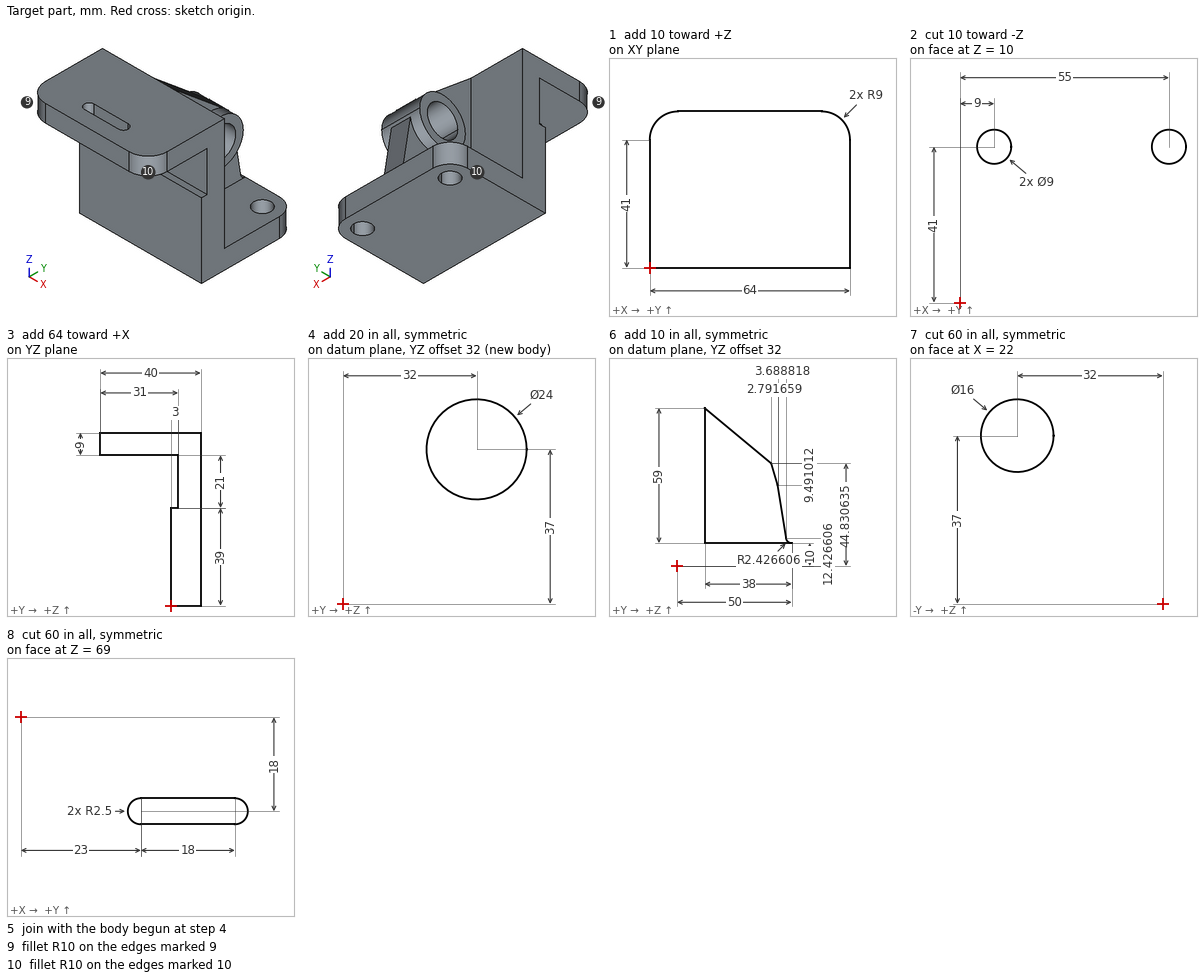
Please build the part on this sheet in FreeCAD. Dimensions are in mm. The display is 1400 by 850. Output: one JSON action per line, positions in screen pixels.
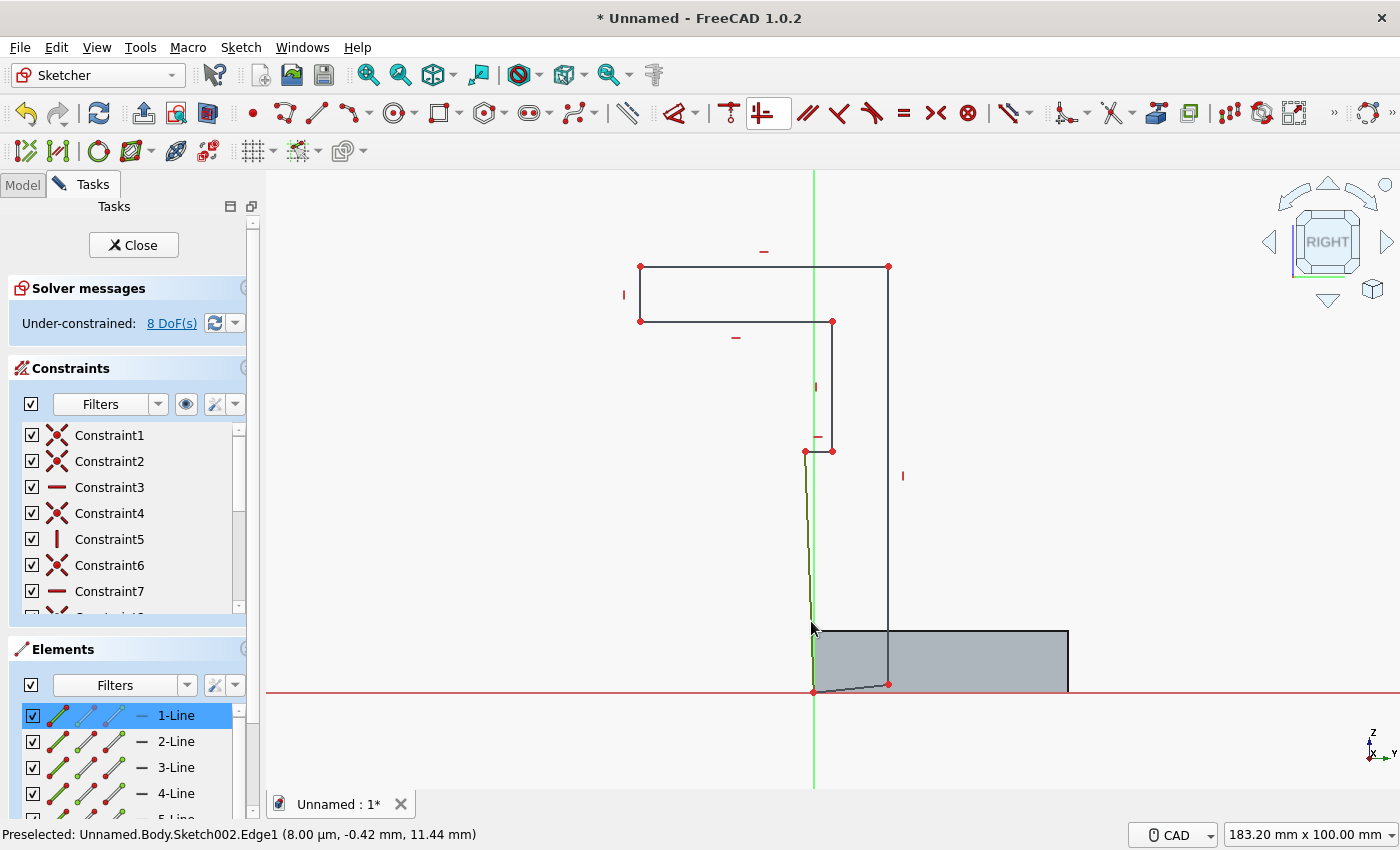
{"action": "key", "text": "v"}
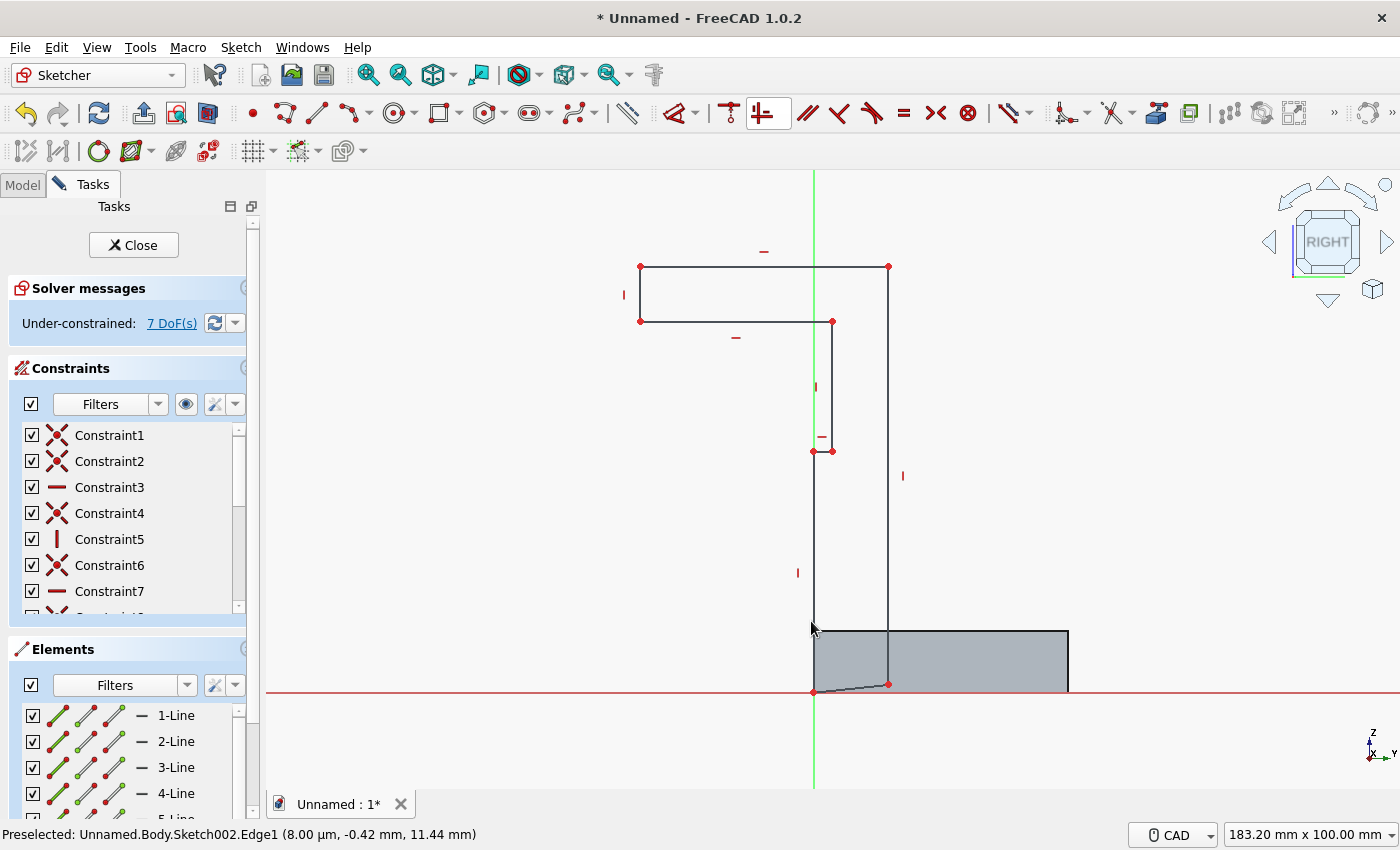
{"action": "left_click", "coordinate": [836, 690]}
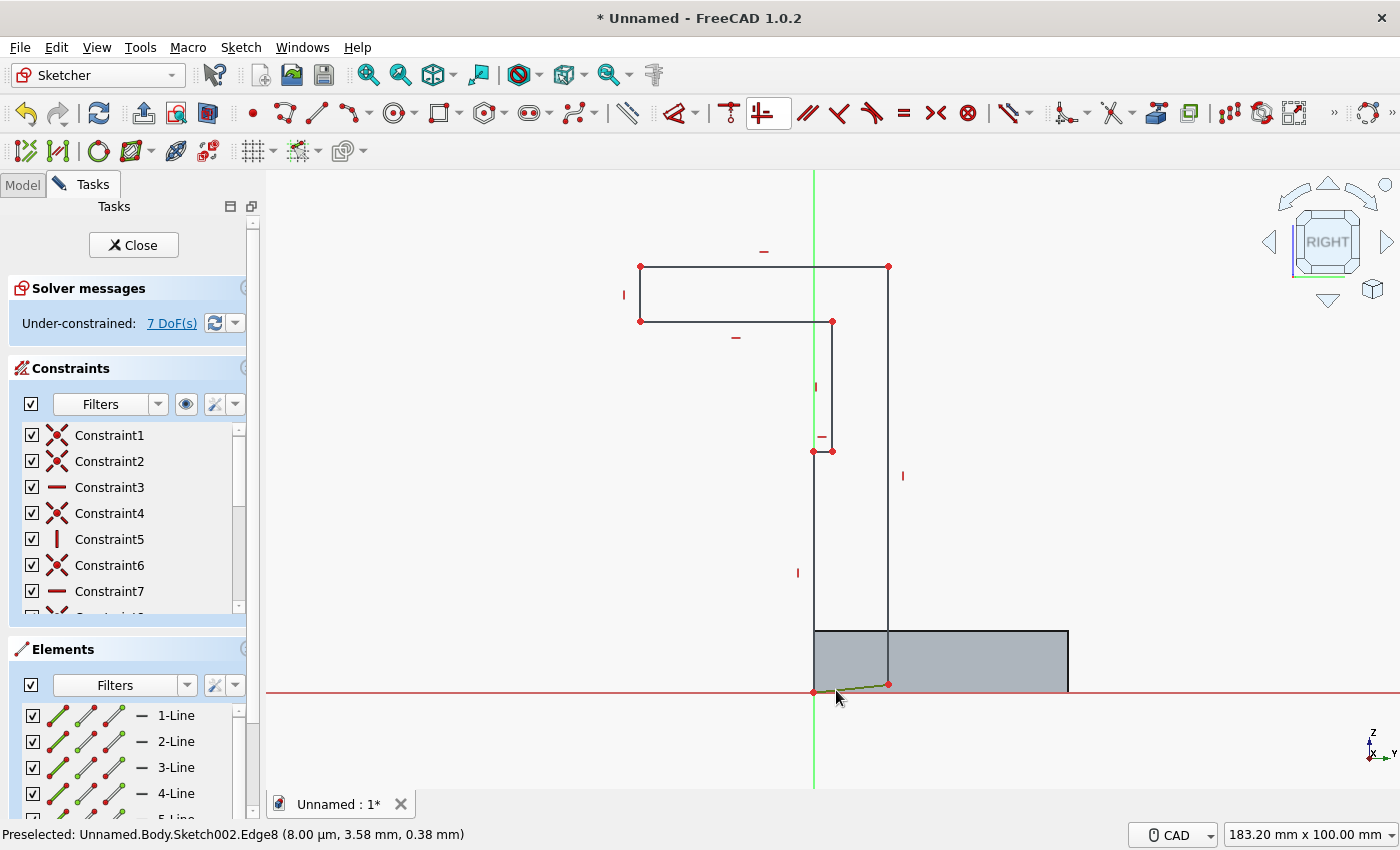
{"action": "key", "text": "h"}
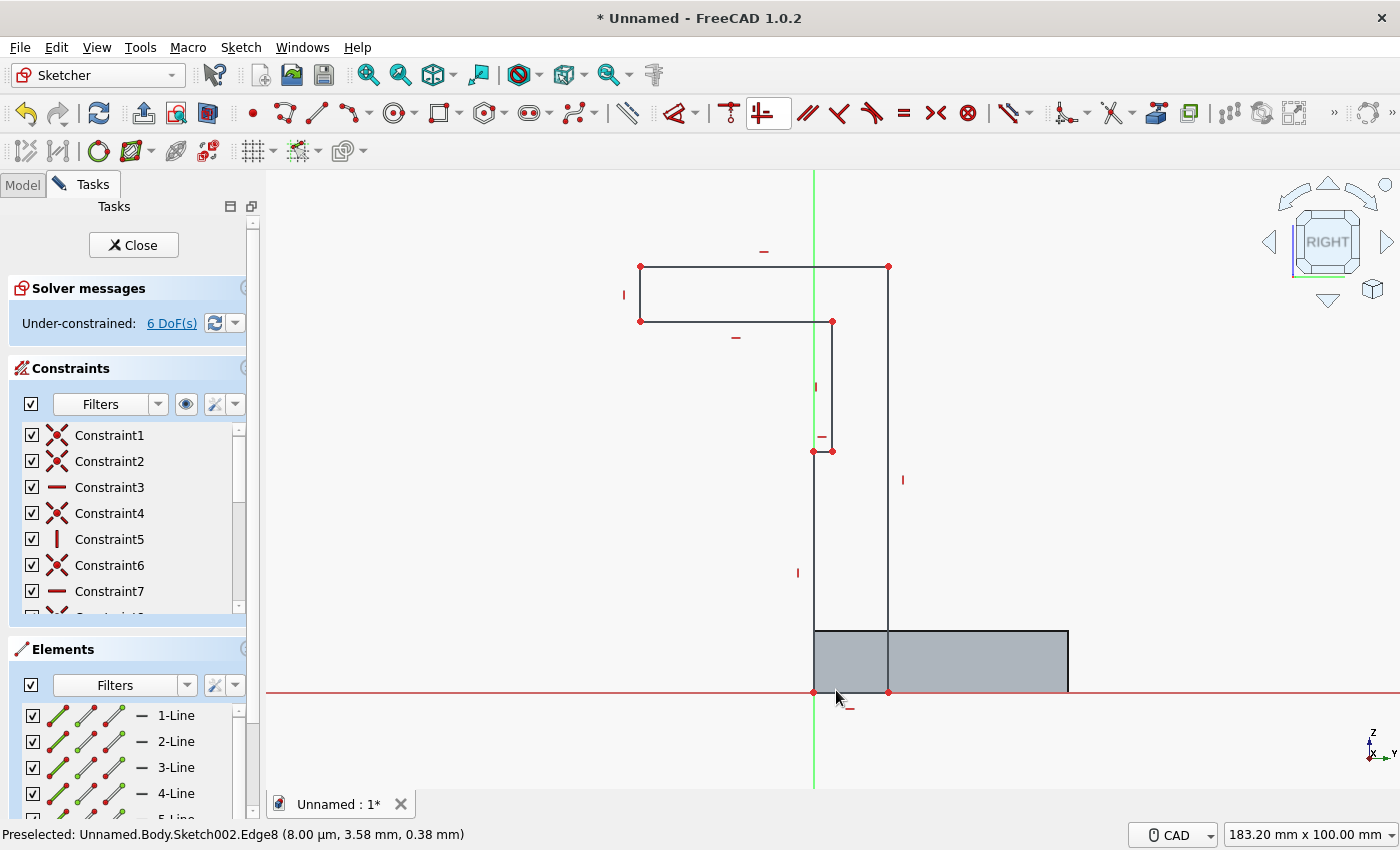
{"action": "left_click", "coordinate": [674, 114]}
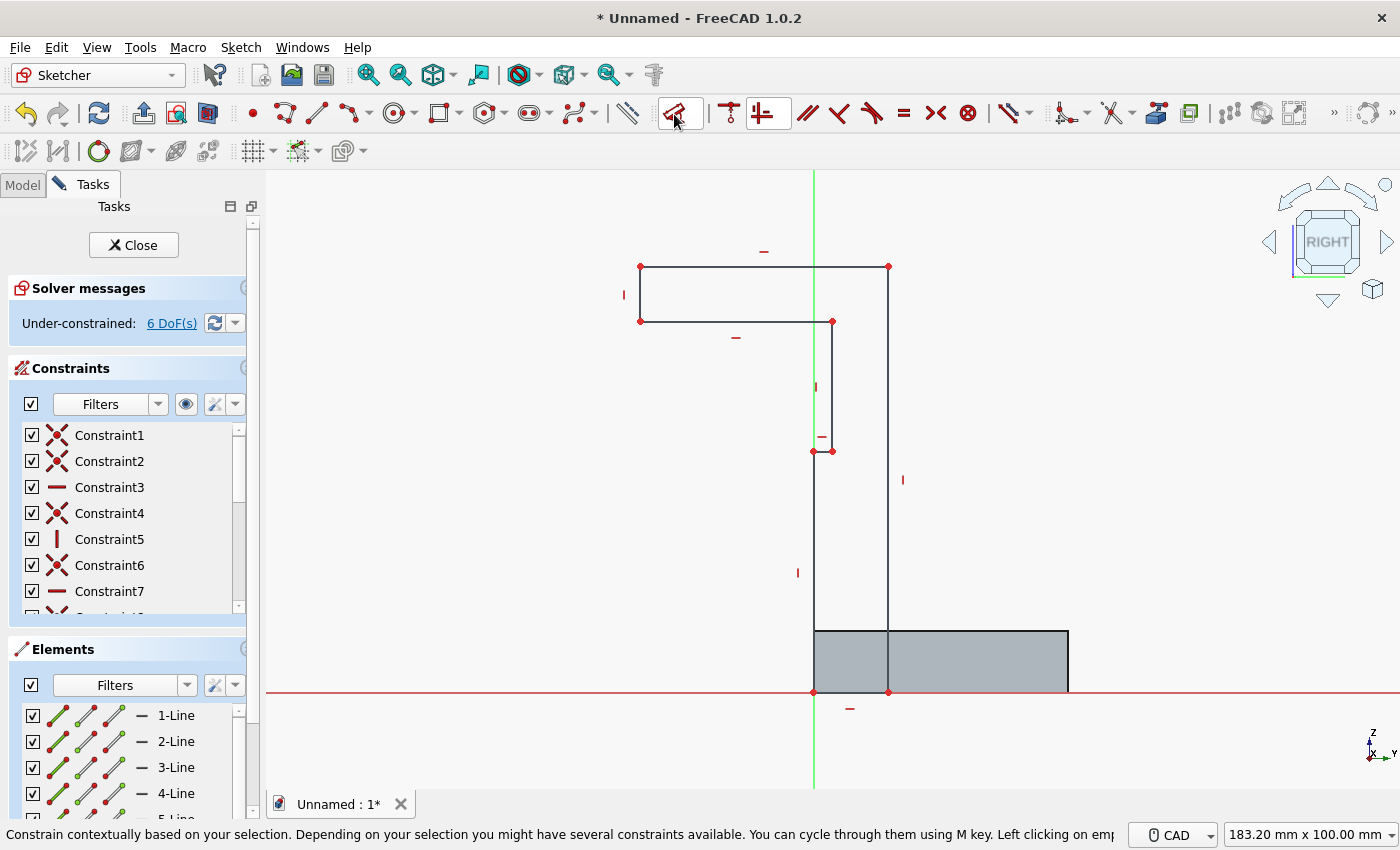
{"action": "scroll", "coordinate": [823, 452], "scroll_direction": "up", "scroll_amount": 4}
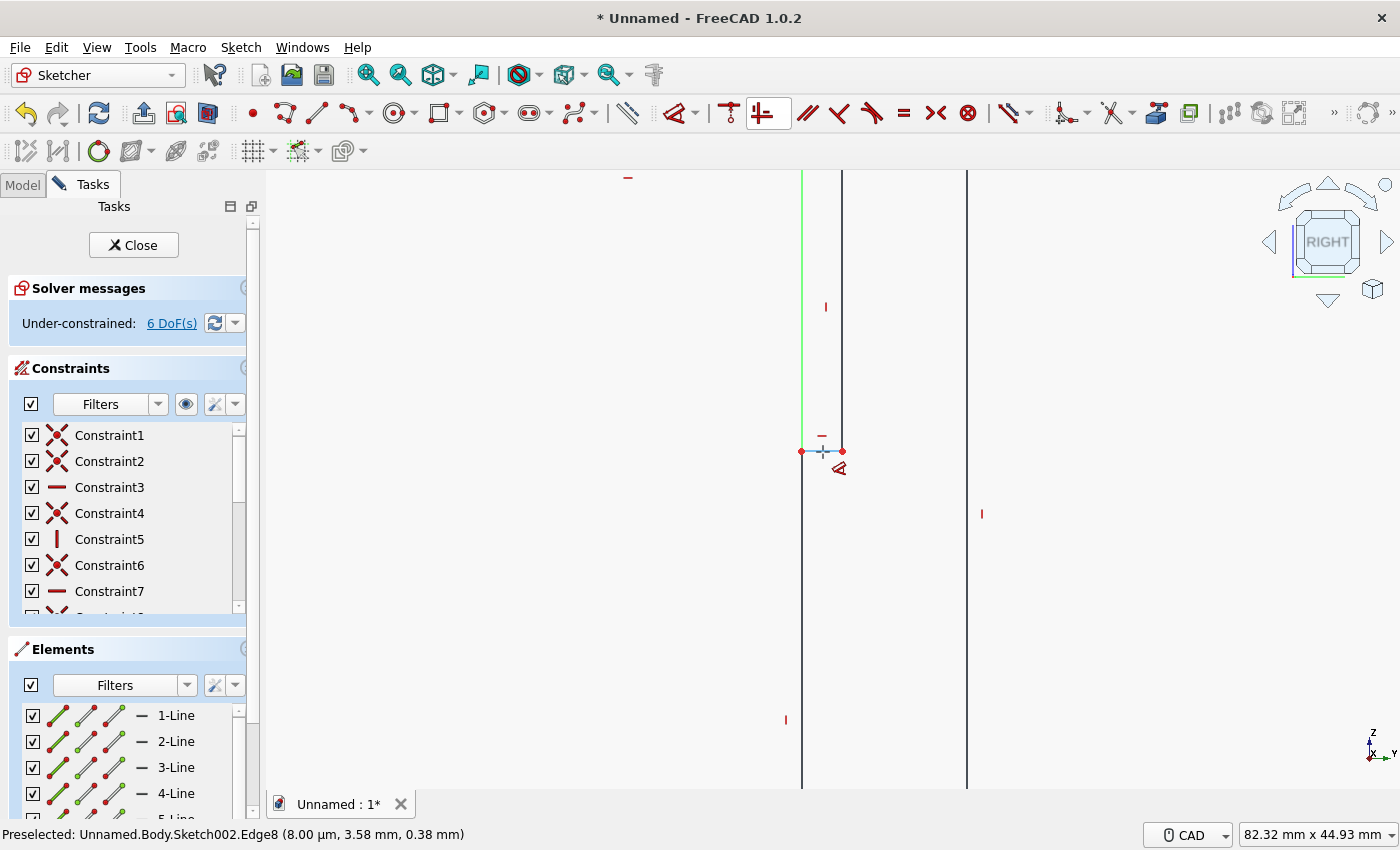
{"action": "left_click", "coordinate": [822, 451]}
{"action": "left_click", "coordinate": [822, 417]}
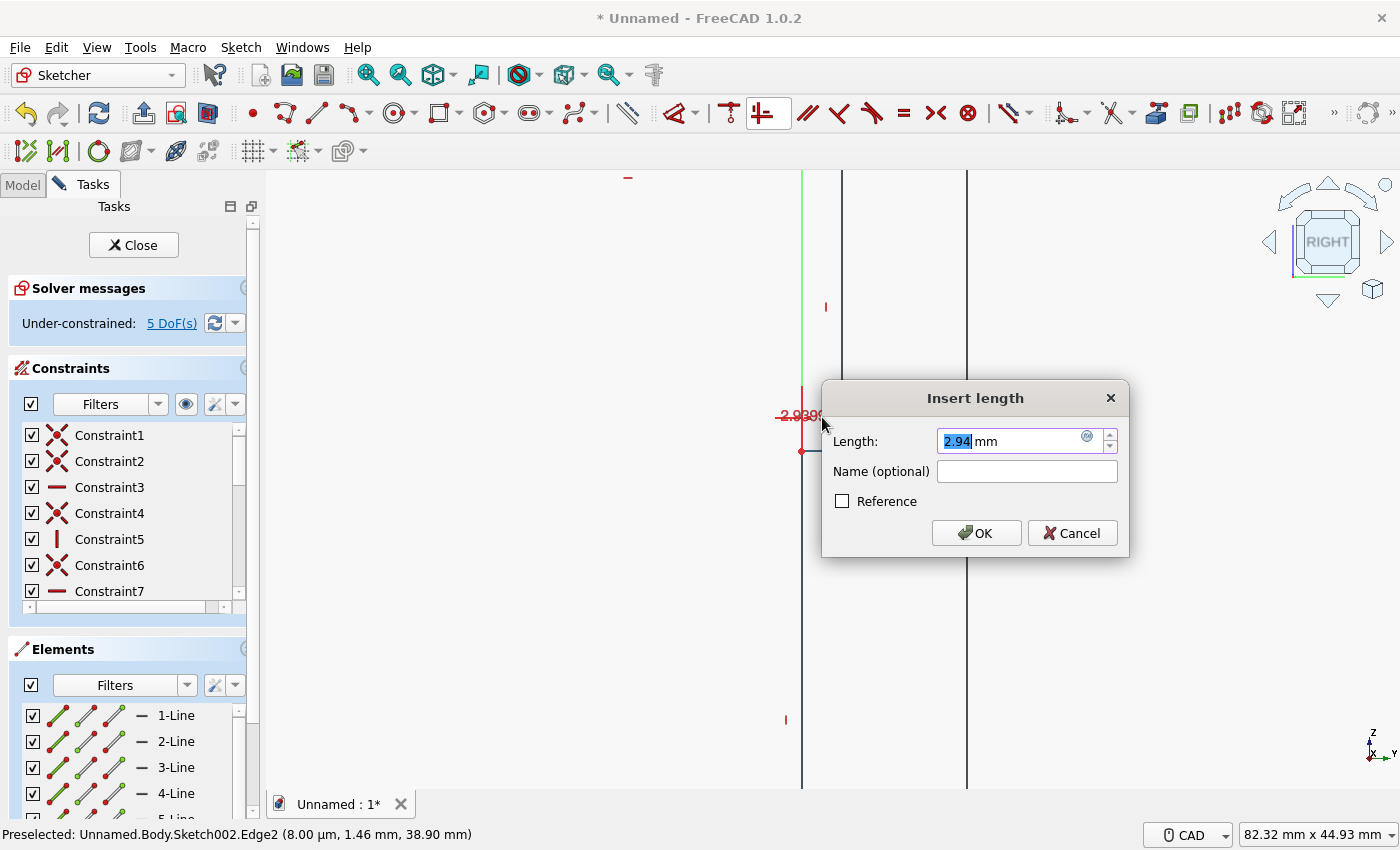
{"action": "type", "text": "3"}
{"action": "key", "text": "Return"}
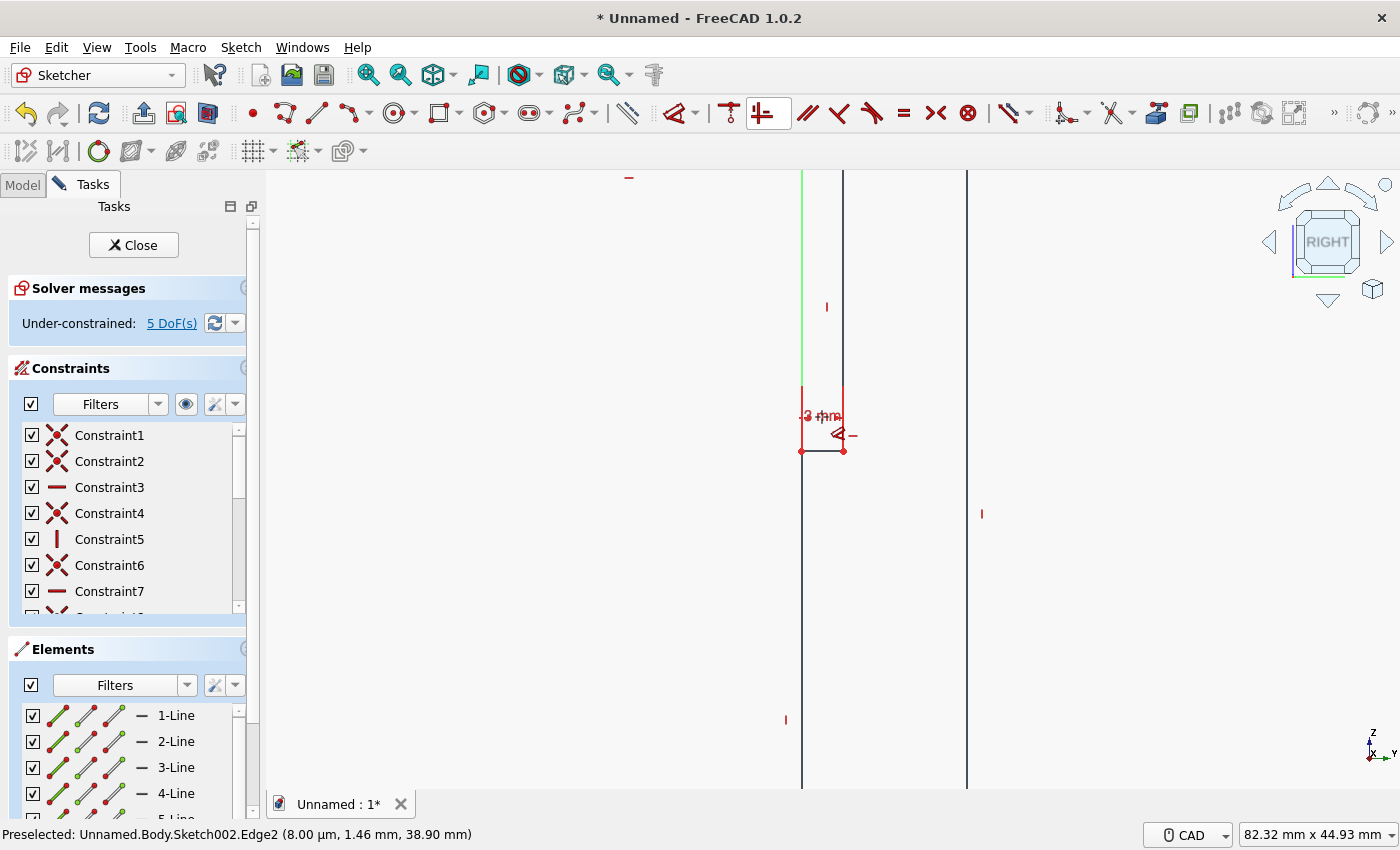
{"action": "scroll", "coordinate": [824, 453], "scroll_direction": "down", "scroll_amount": 4}